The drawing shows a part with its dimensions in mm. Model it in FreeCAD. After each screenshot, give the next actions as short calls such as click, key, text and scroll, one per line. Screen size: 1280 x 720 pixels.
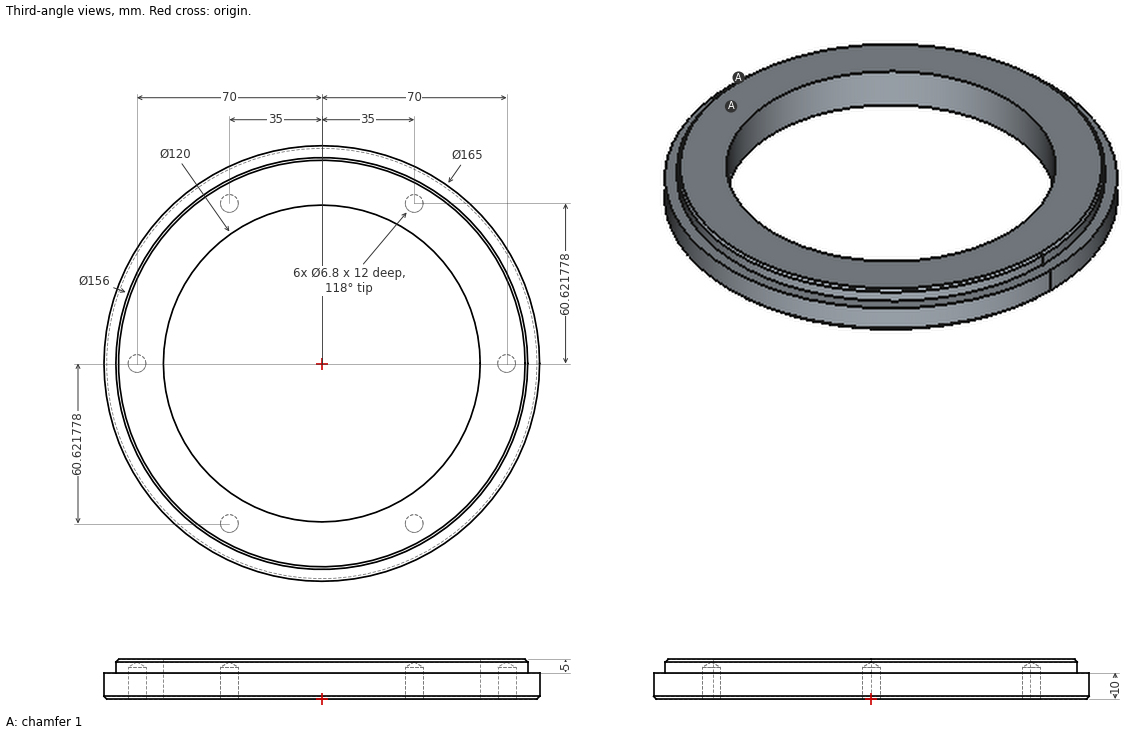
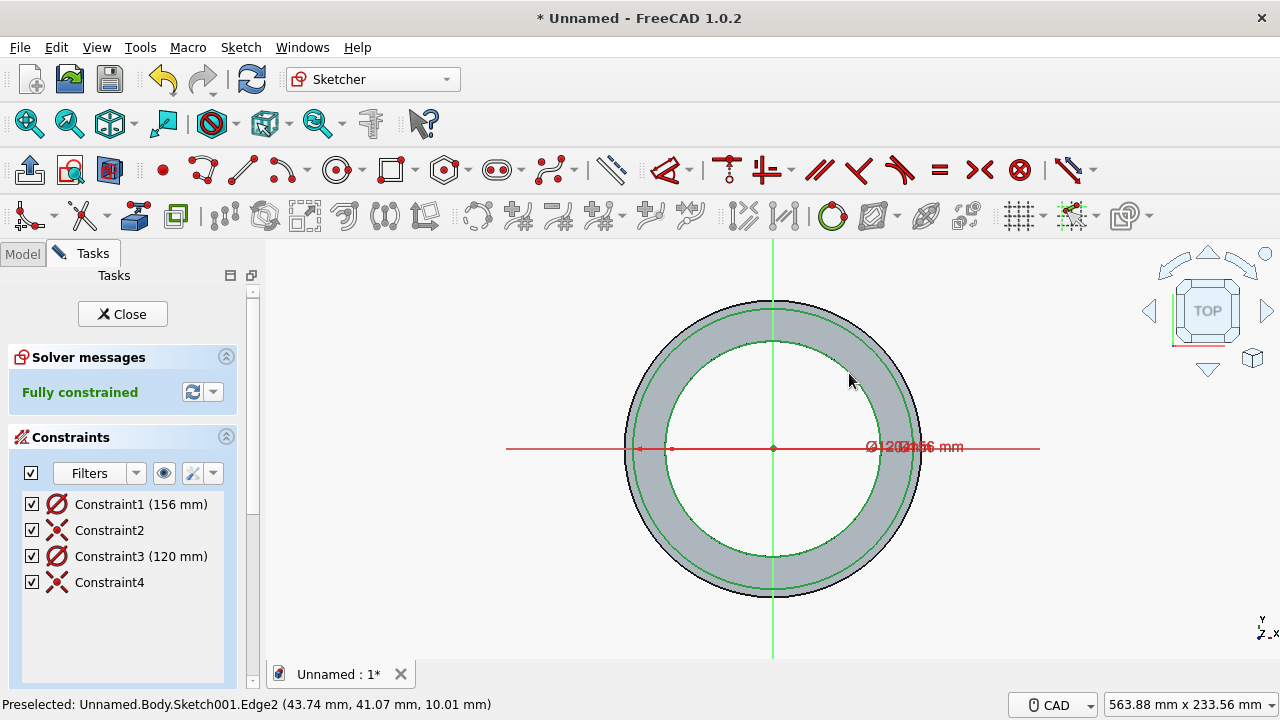
click(123, 314)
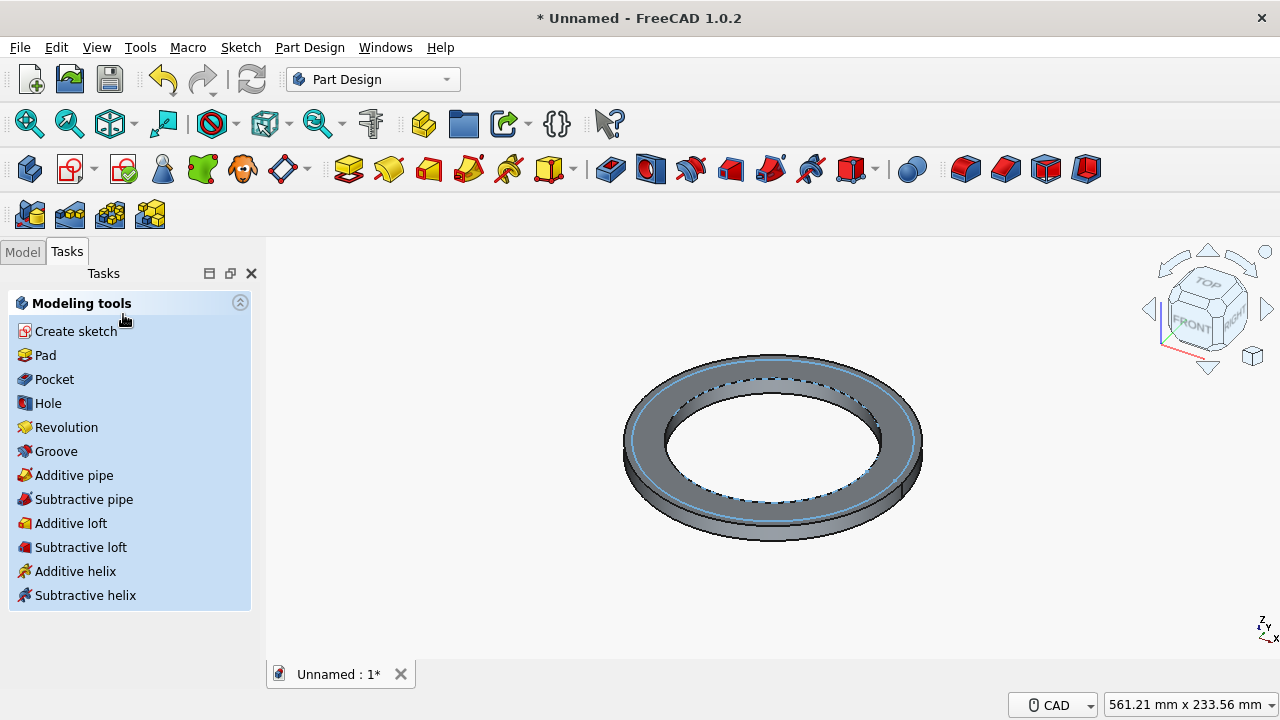
click(350, 170)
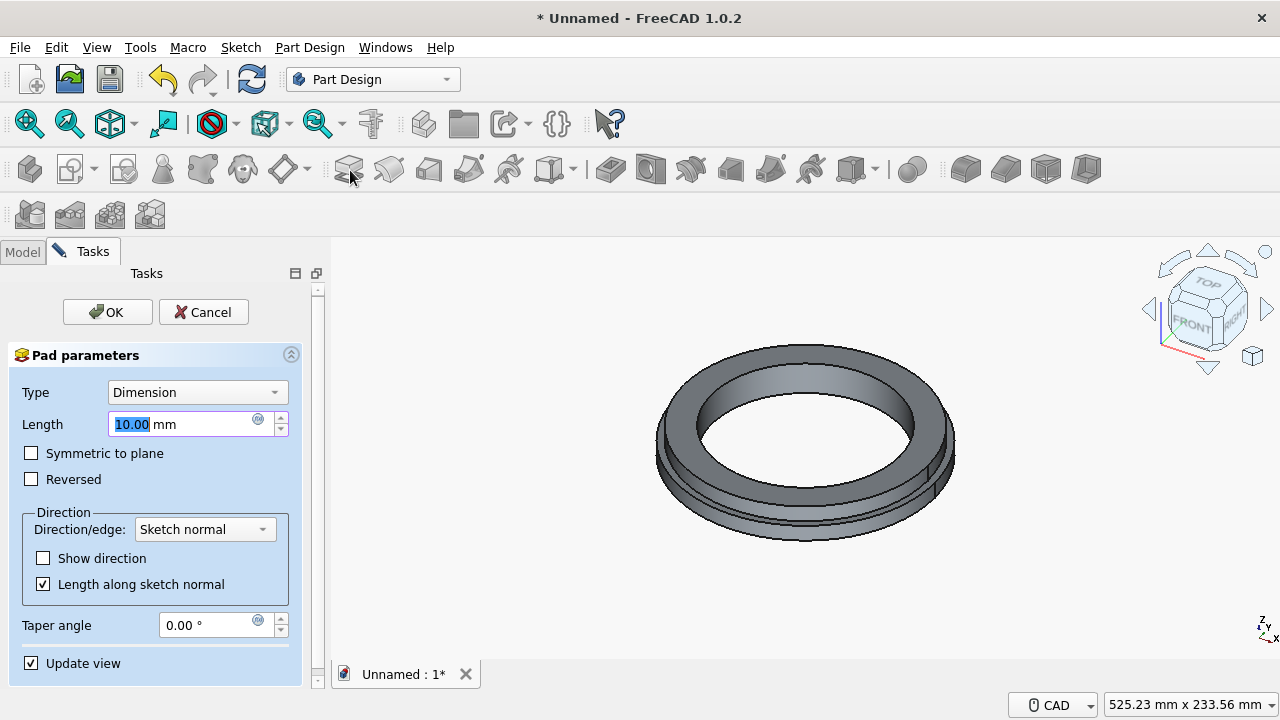
text(5)
key(Tab)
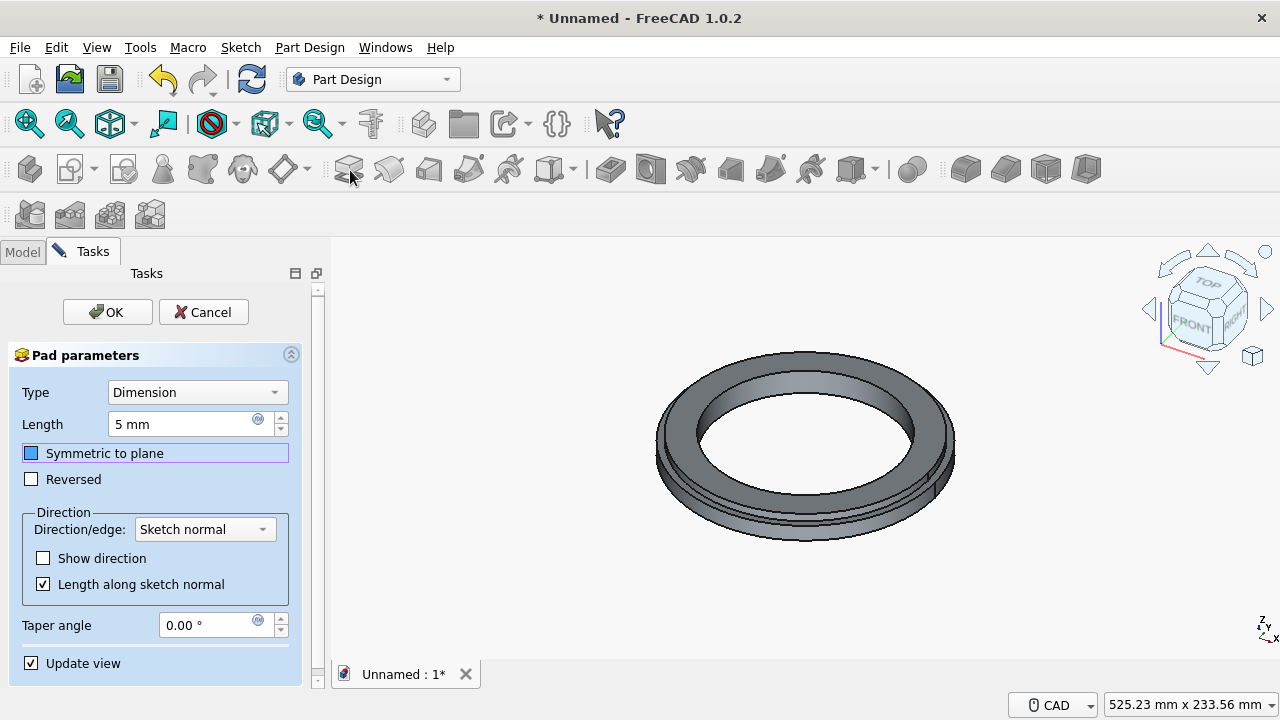
click(108, 312)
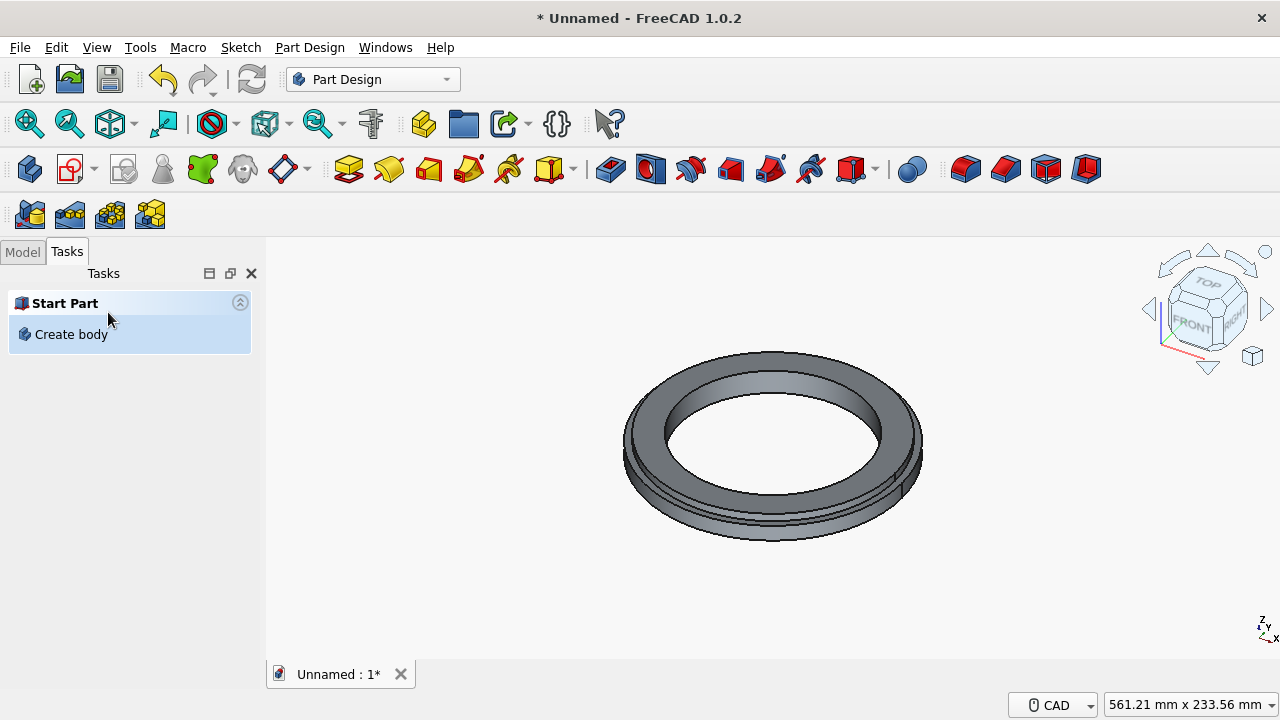
click(633, 440)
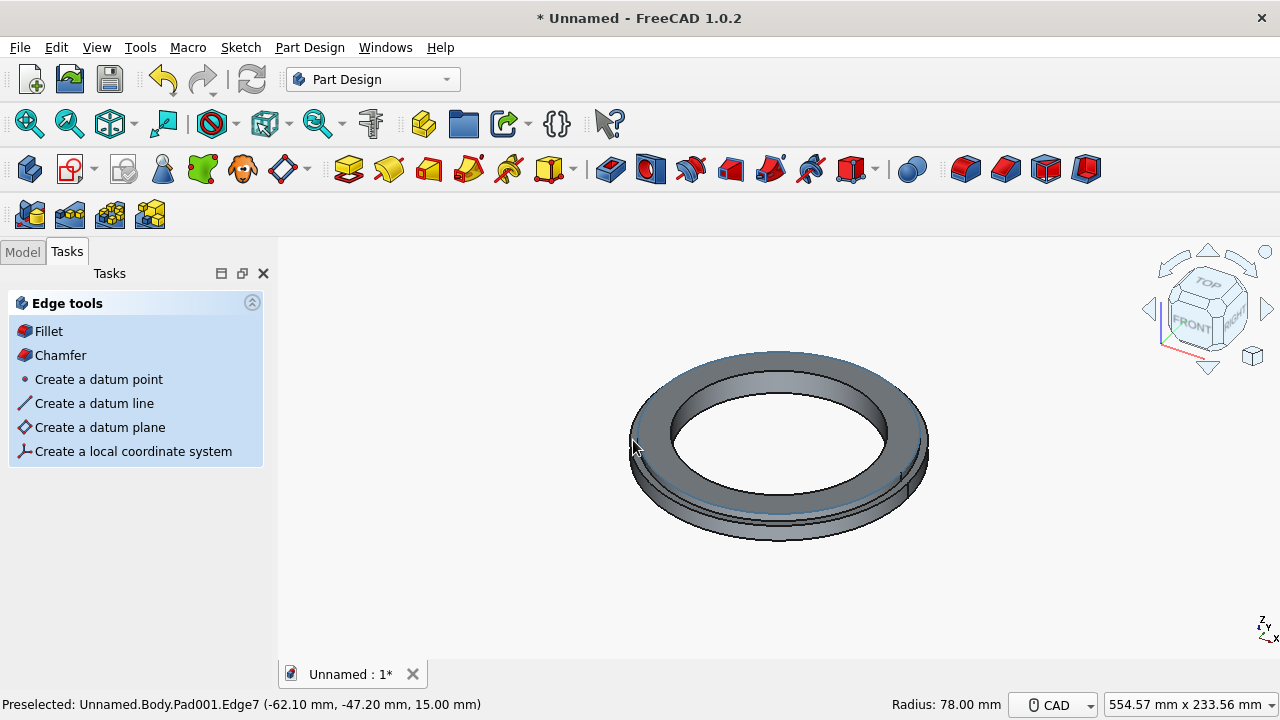
key(0)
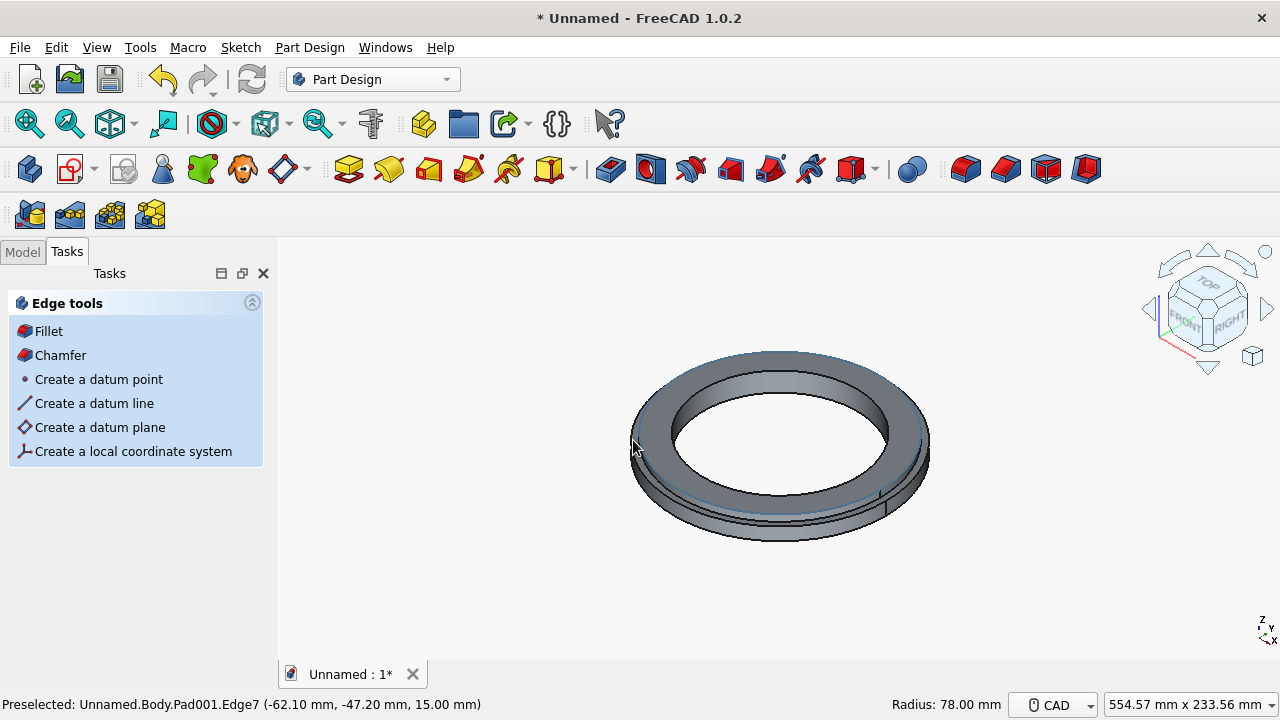
key(2)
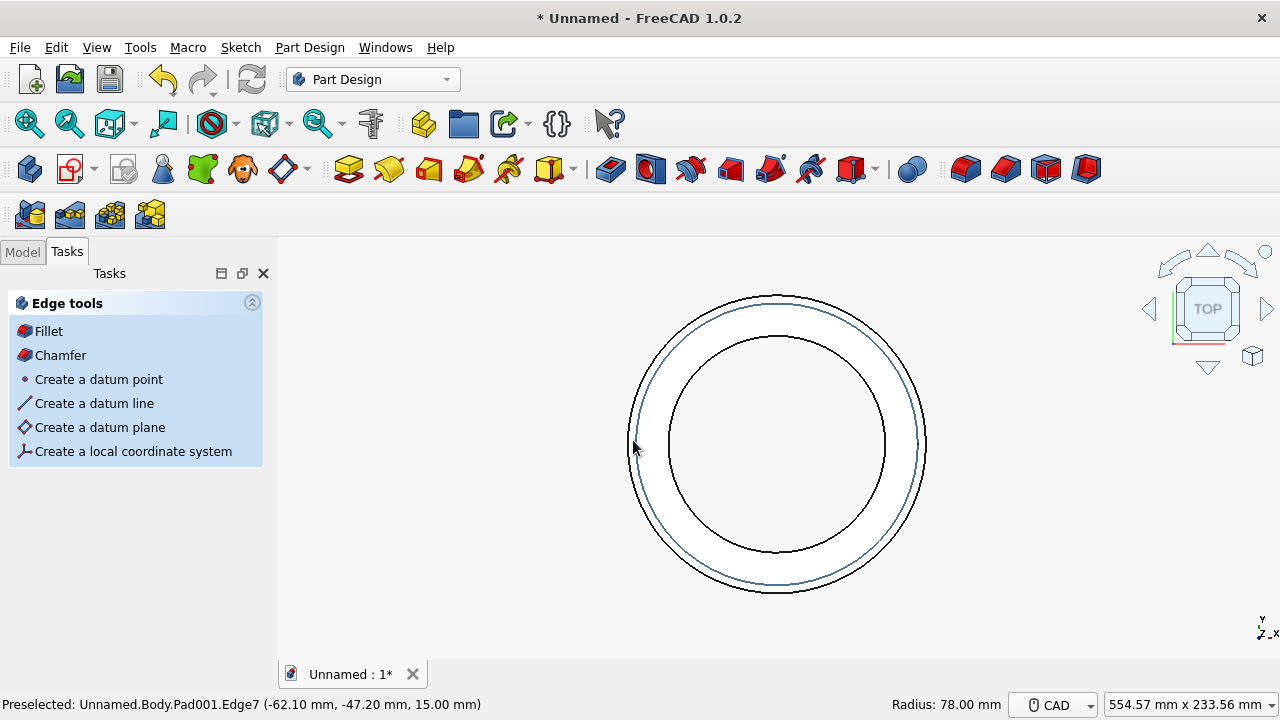
key(1)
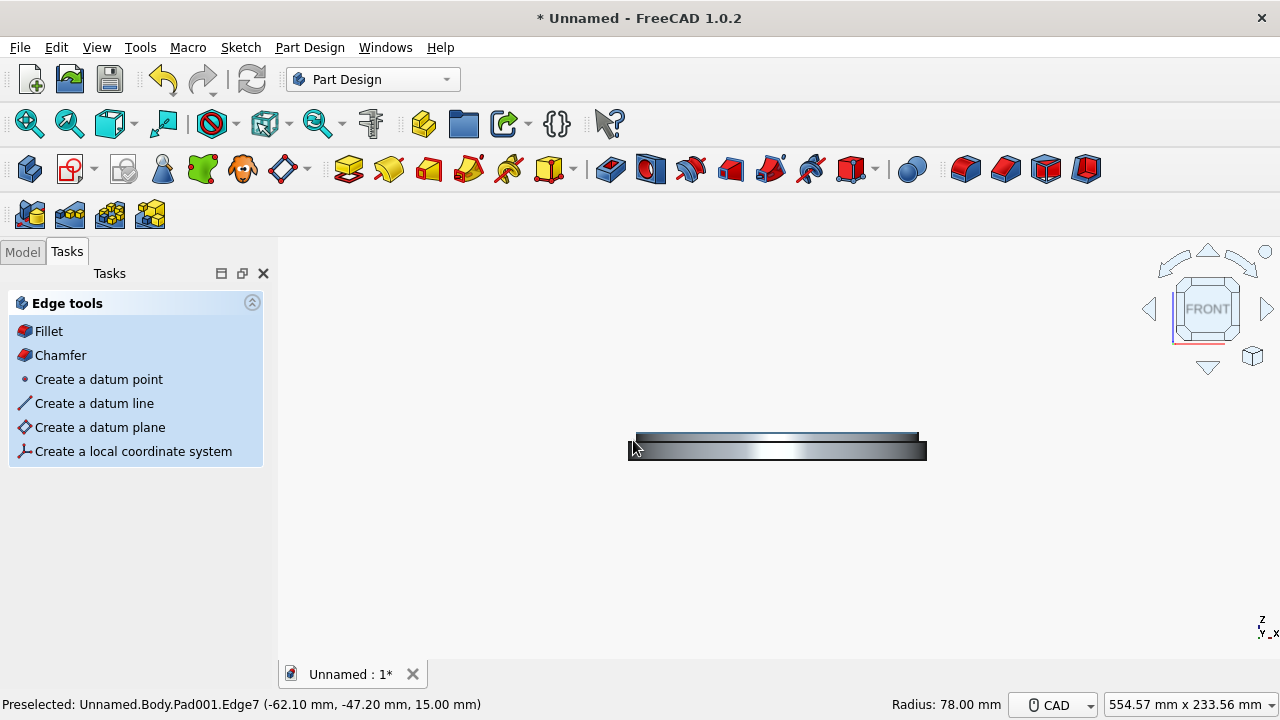
click(30, 124)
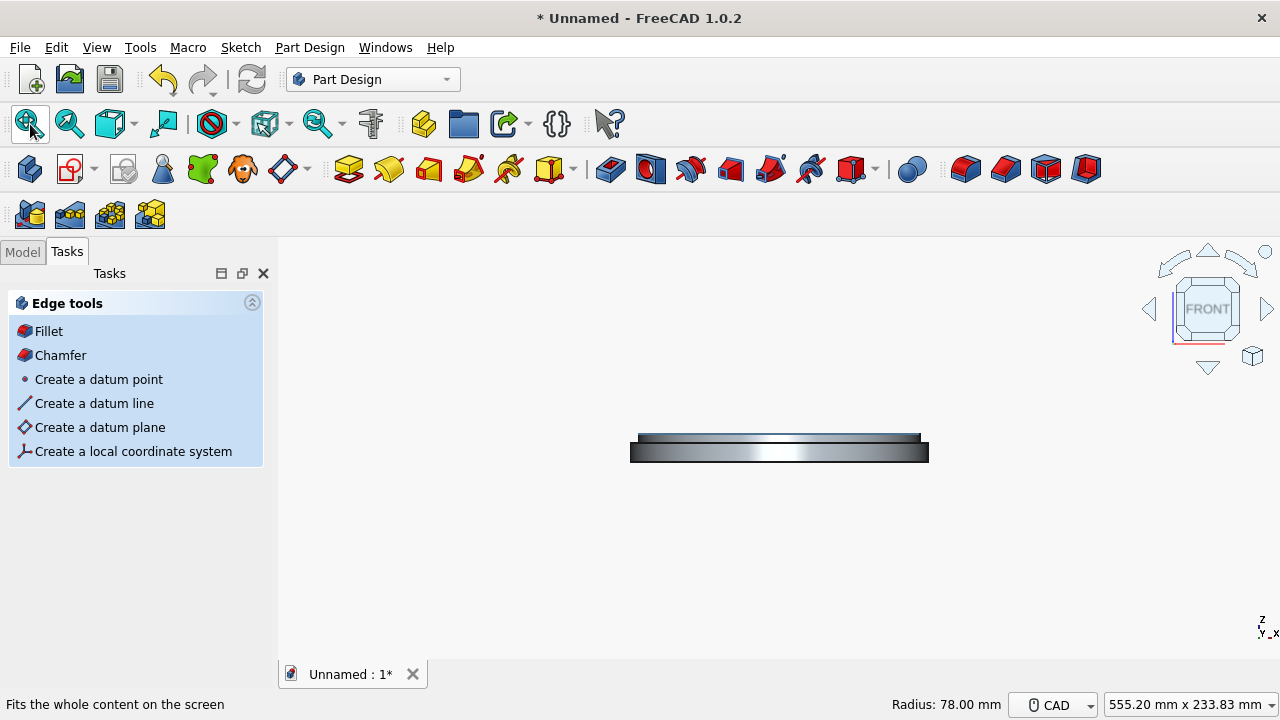
click(659, 461, ctrl)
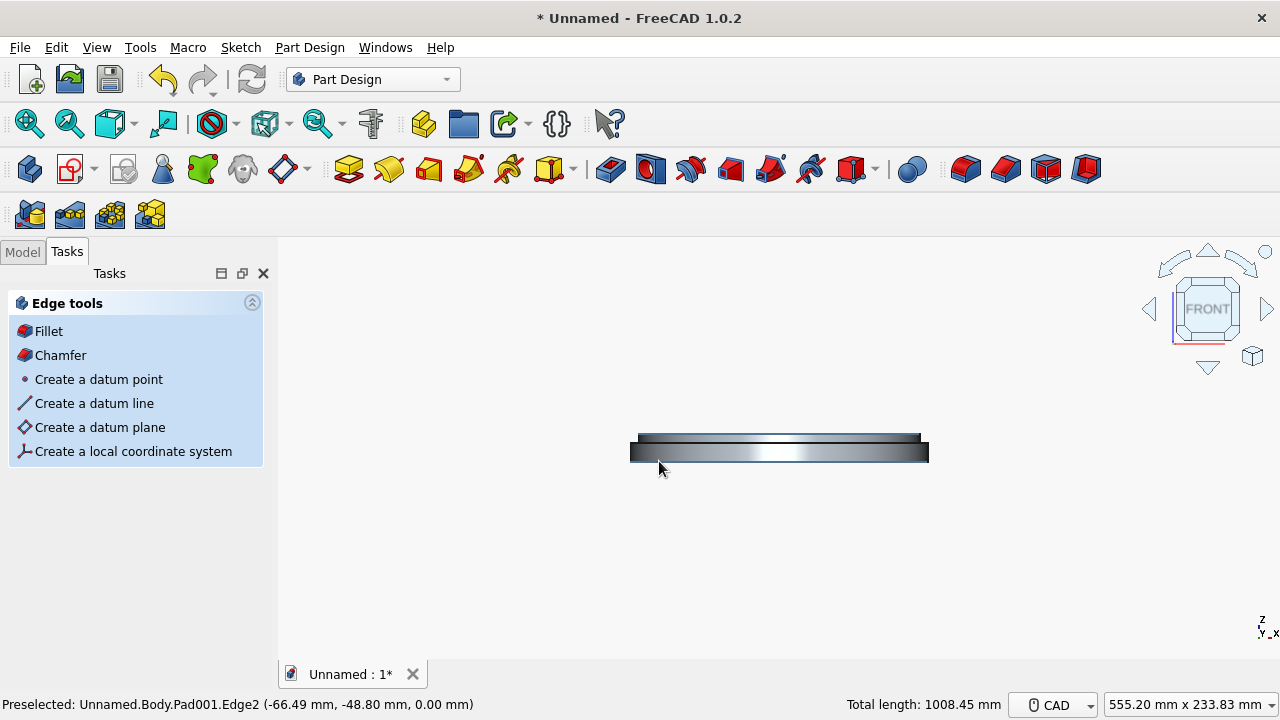
click(1006, 170)